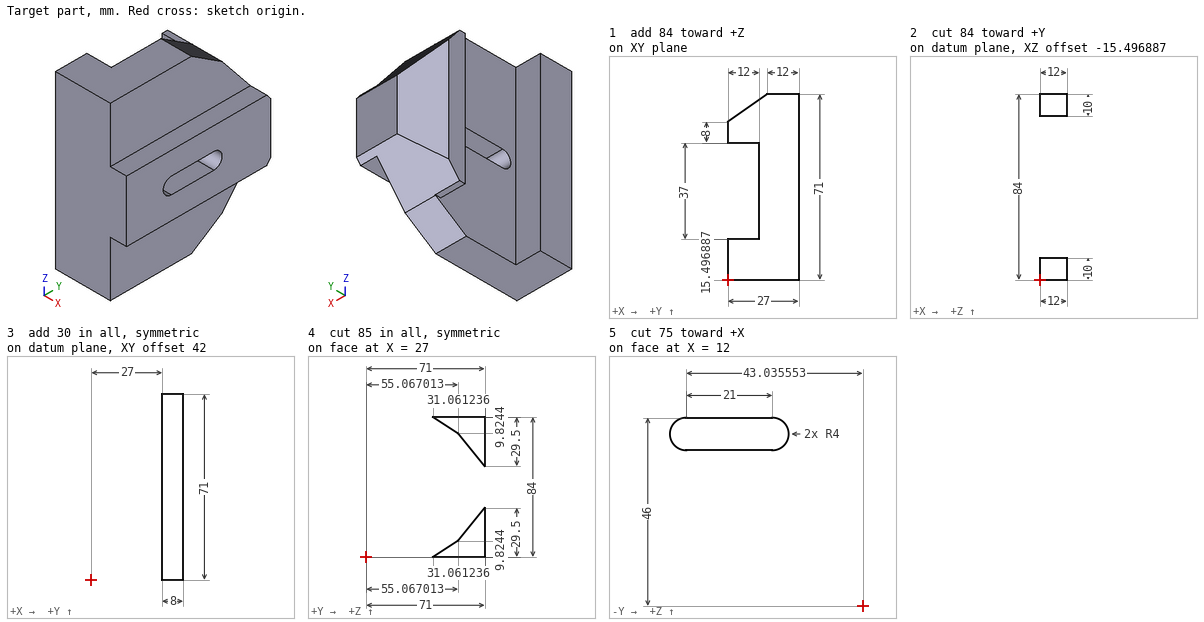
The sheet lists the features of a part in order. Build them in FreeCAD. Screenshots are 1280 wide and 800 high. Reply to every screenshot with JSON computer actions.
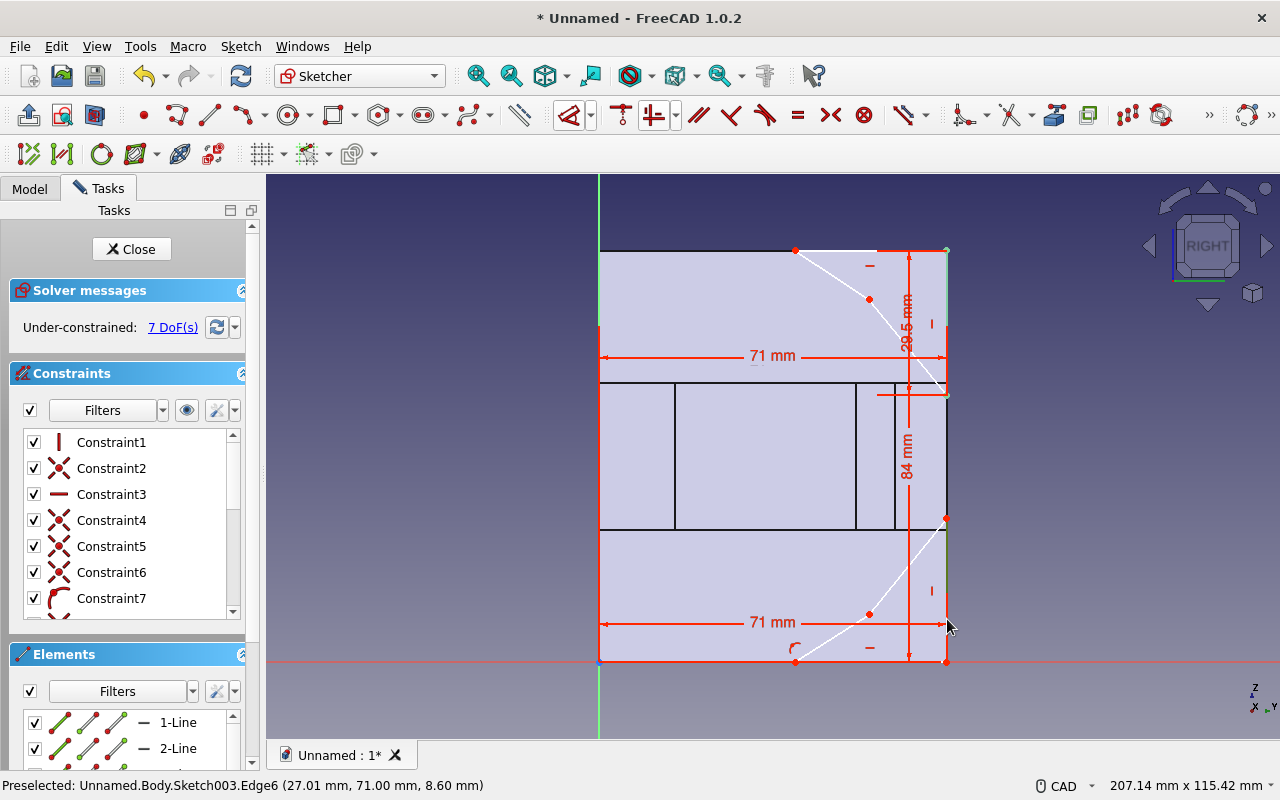
{"action": "key", "text": "i"}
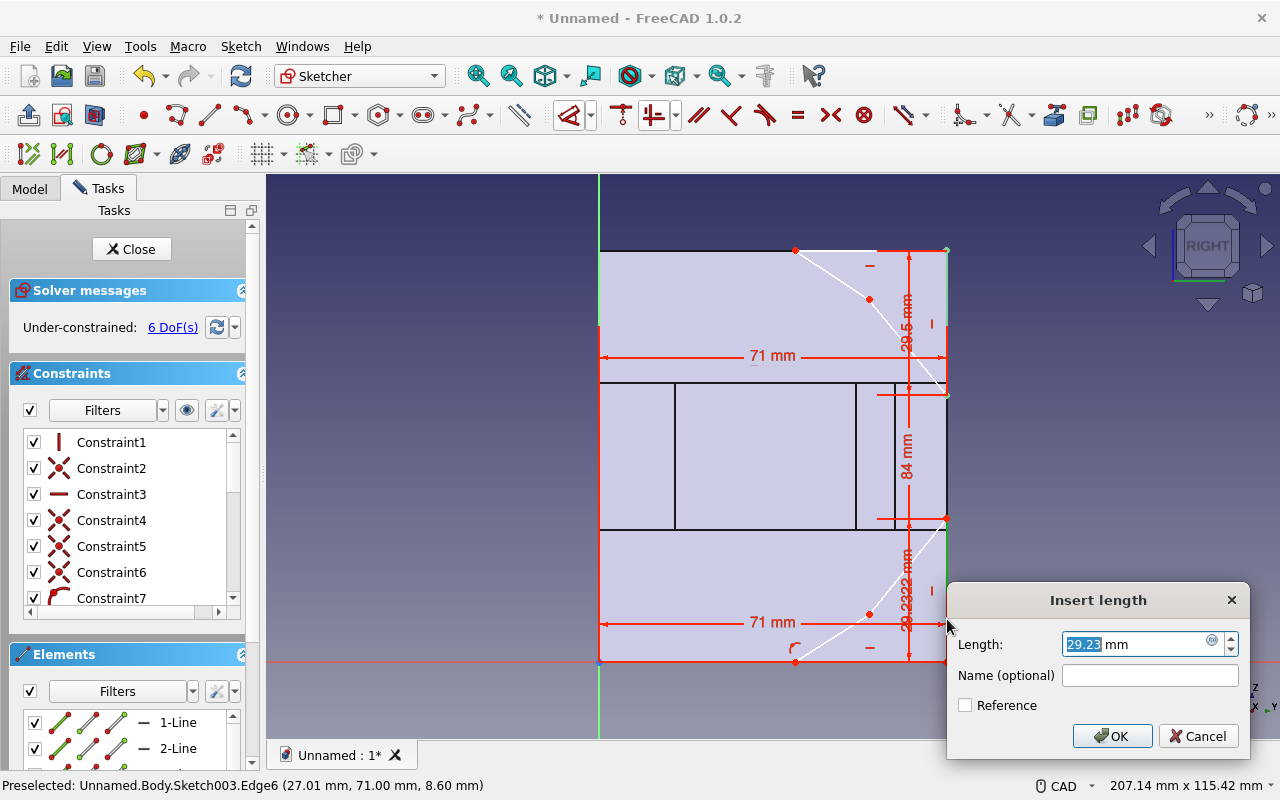
{"action": "type", "text": "29.5"}
{"action": "key", "text": "Return"}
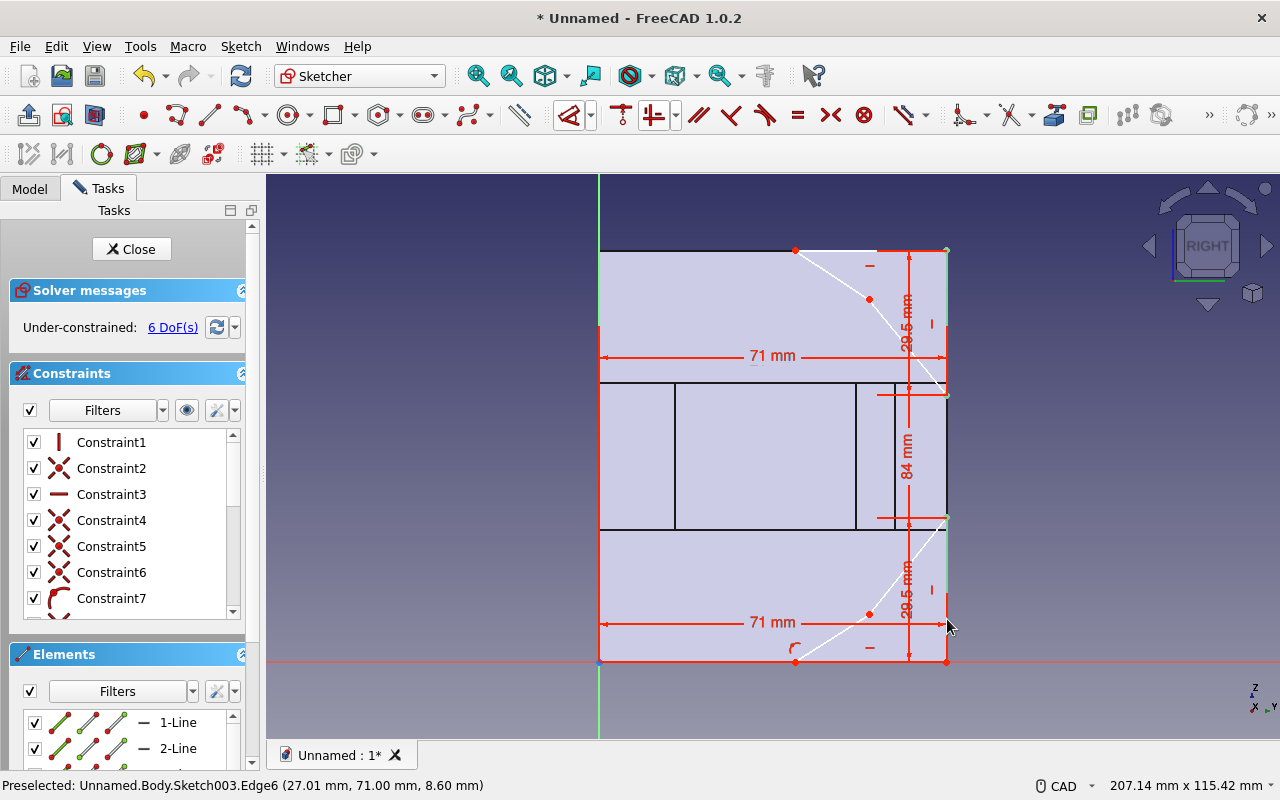
{"action": "left_click", "coordinate": [869, 615]}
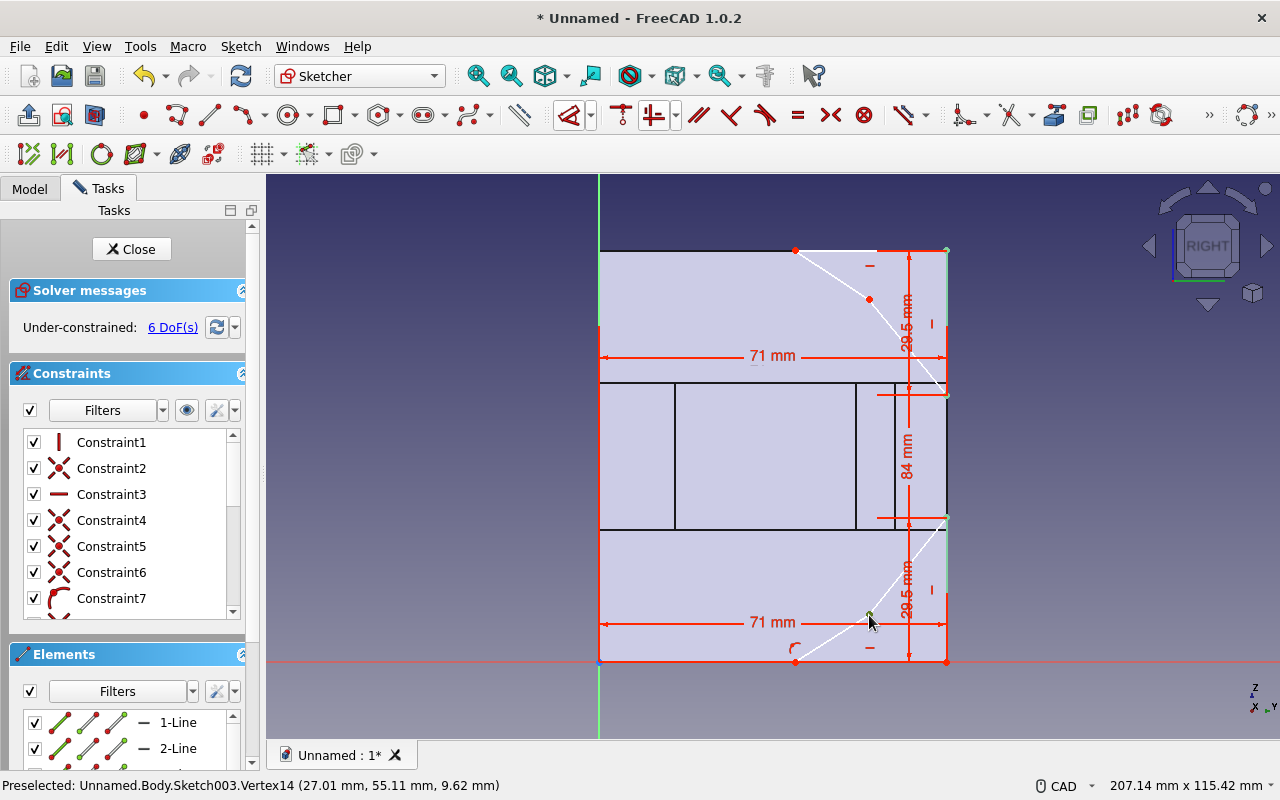
{"action": "left_click", "coordinate": [590, 116]}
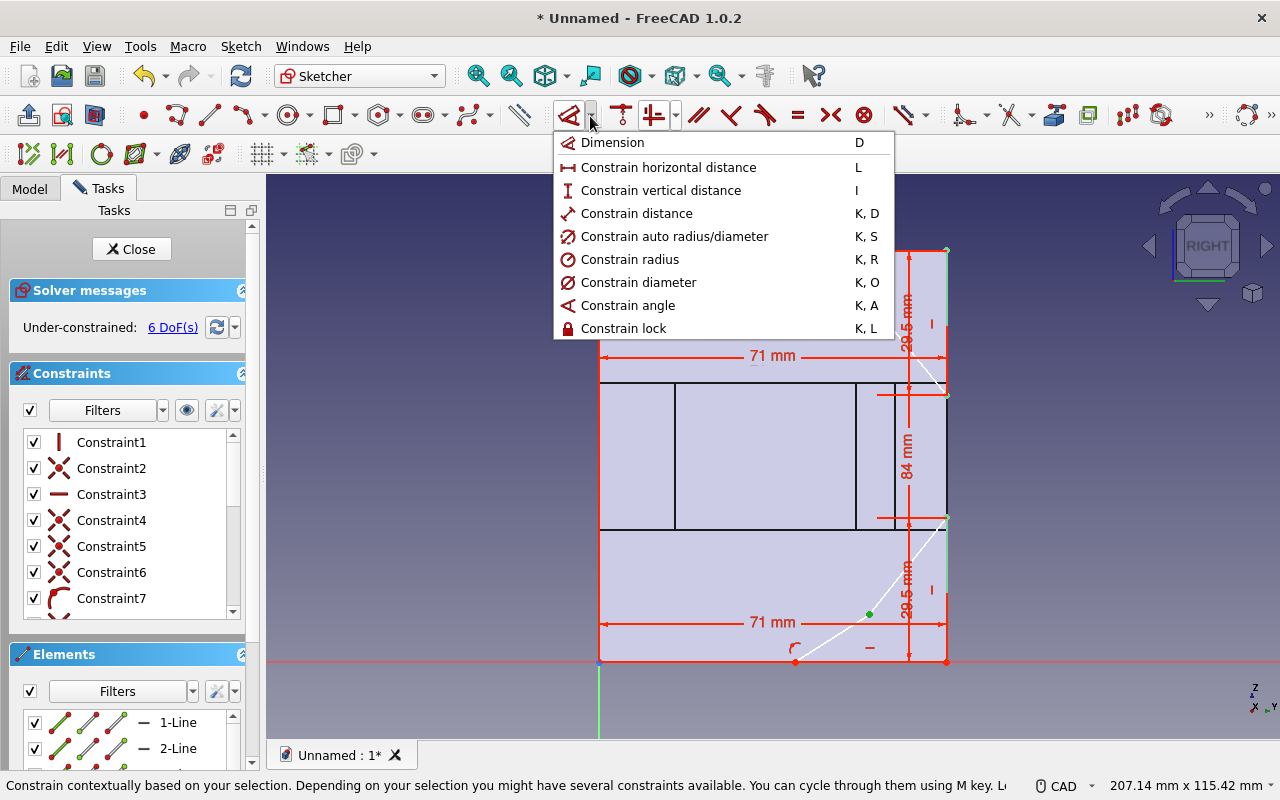
{"action": "left_click", "coordinate": [724, 190]}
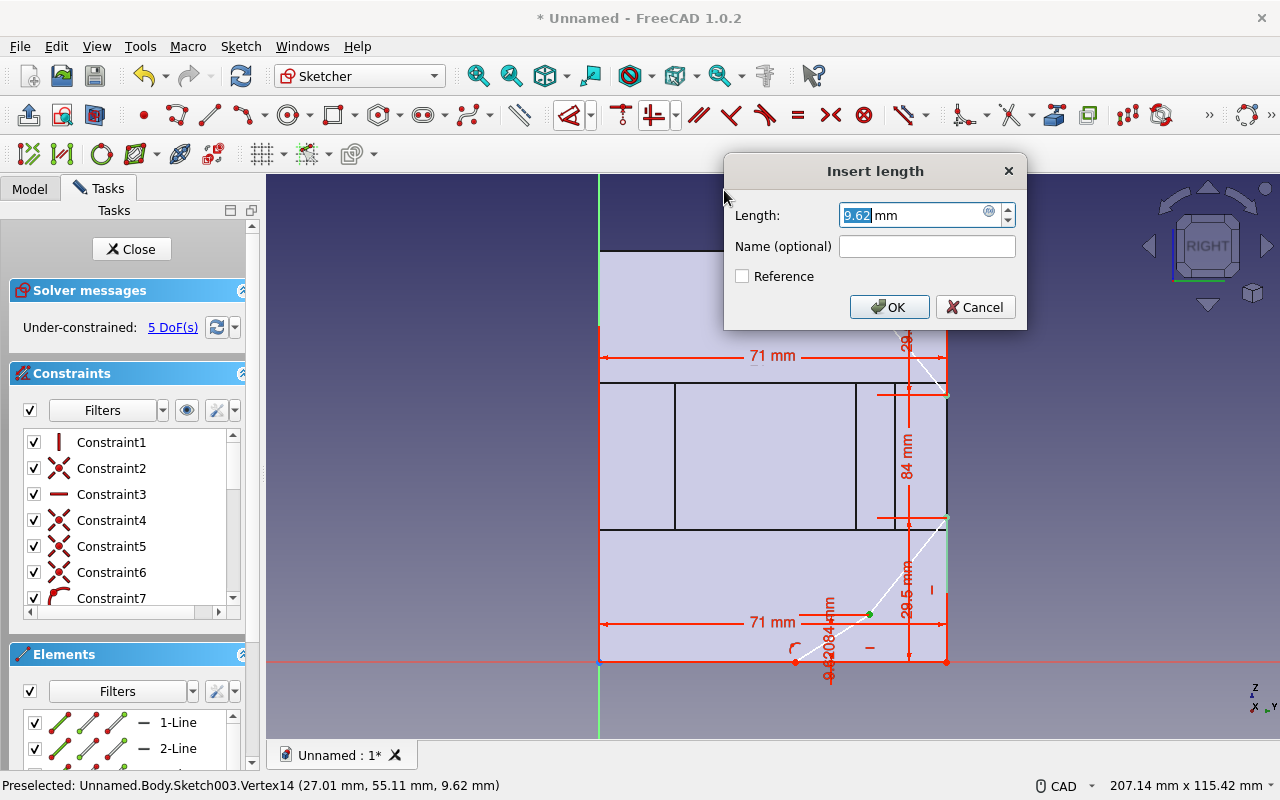
{"action": "type", "text": "9.8244"}
{"action": "key", "text": "Return"}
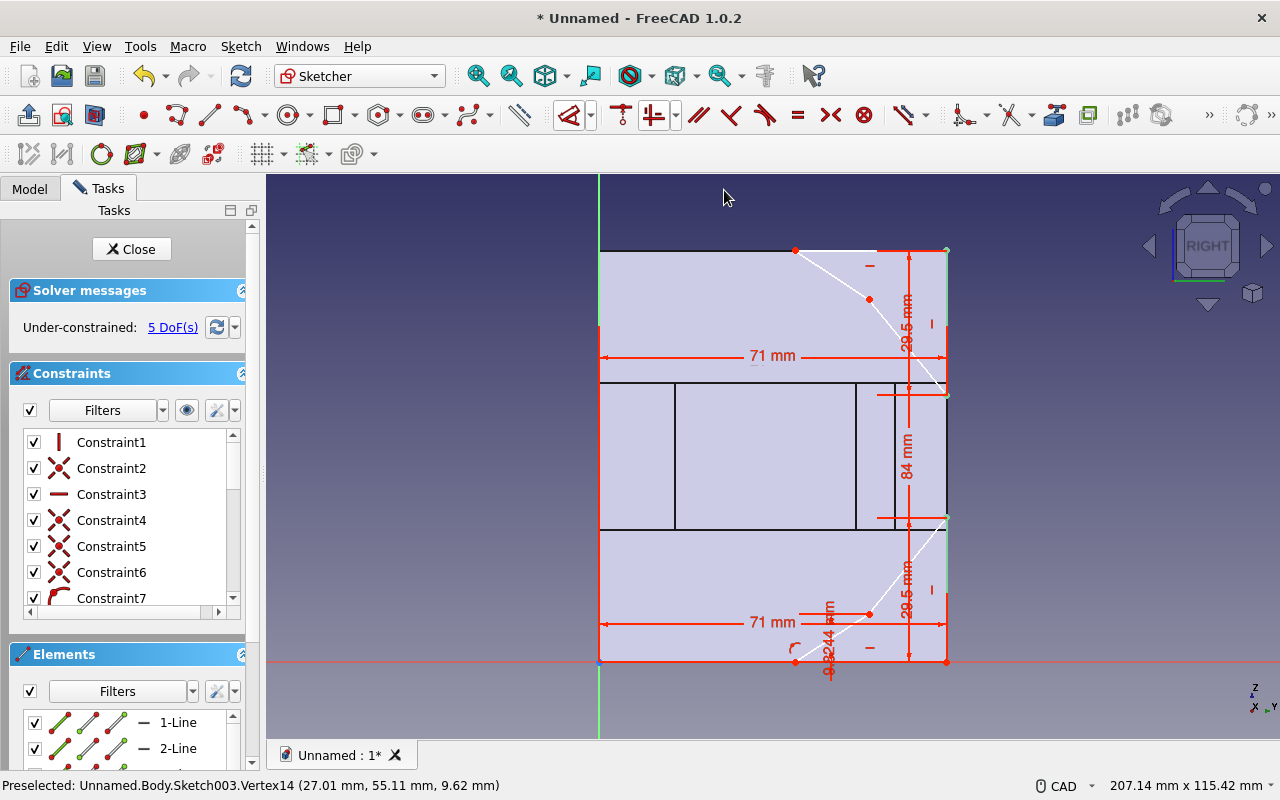
{"action": "left_click", "coordinate": [817, 266]}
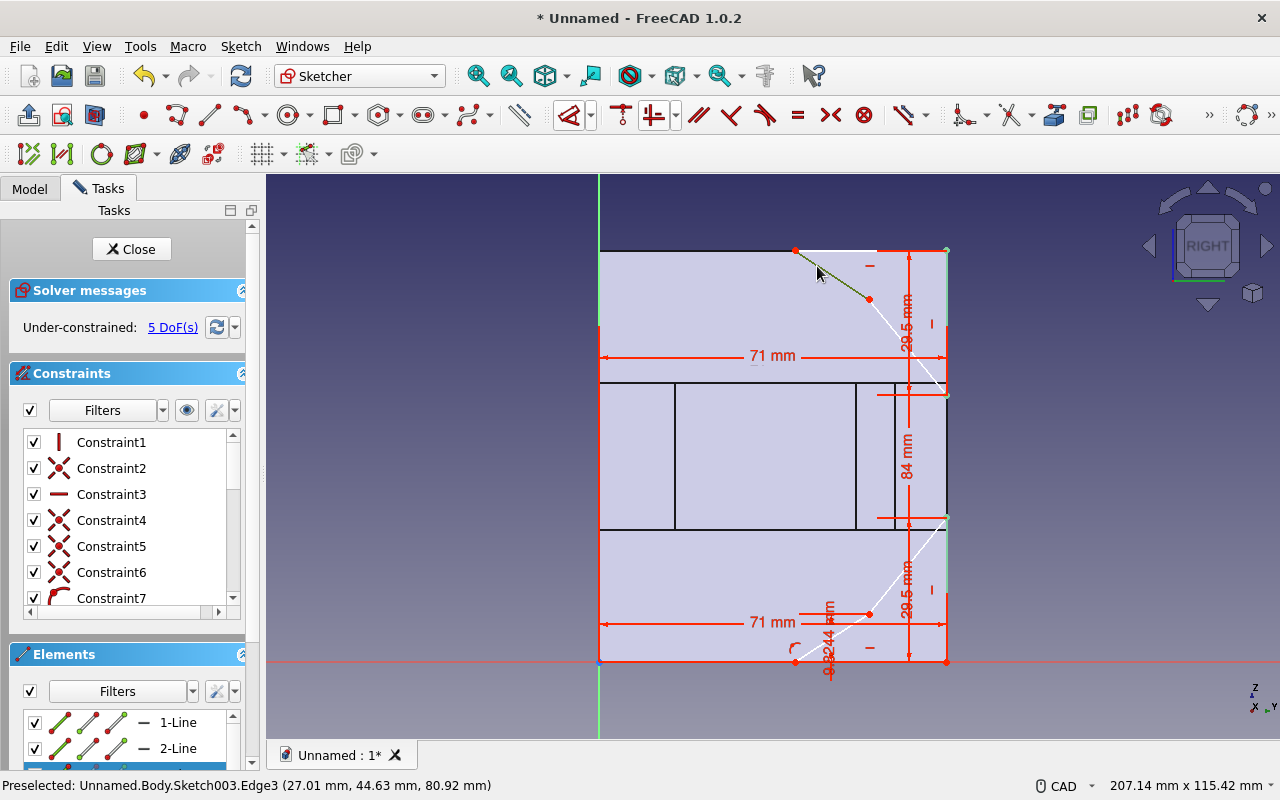
{"action": "left_click", "coordinate": [590, 116]}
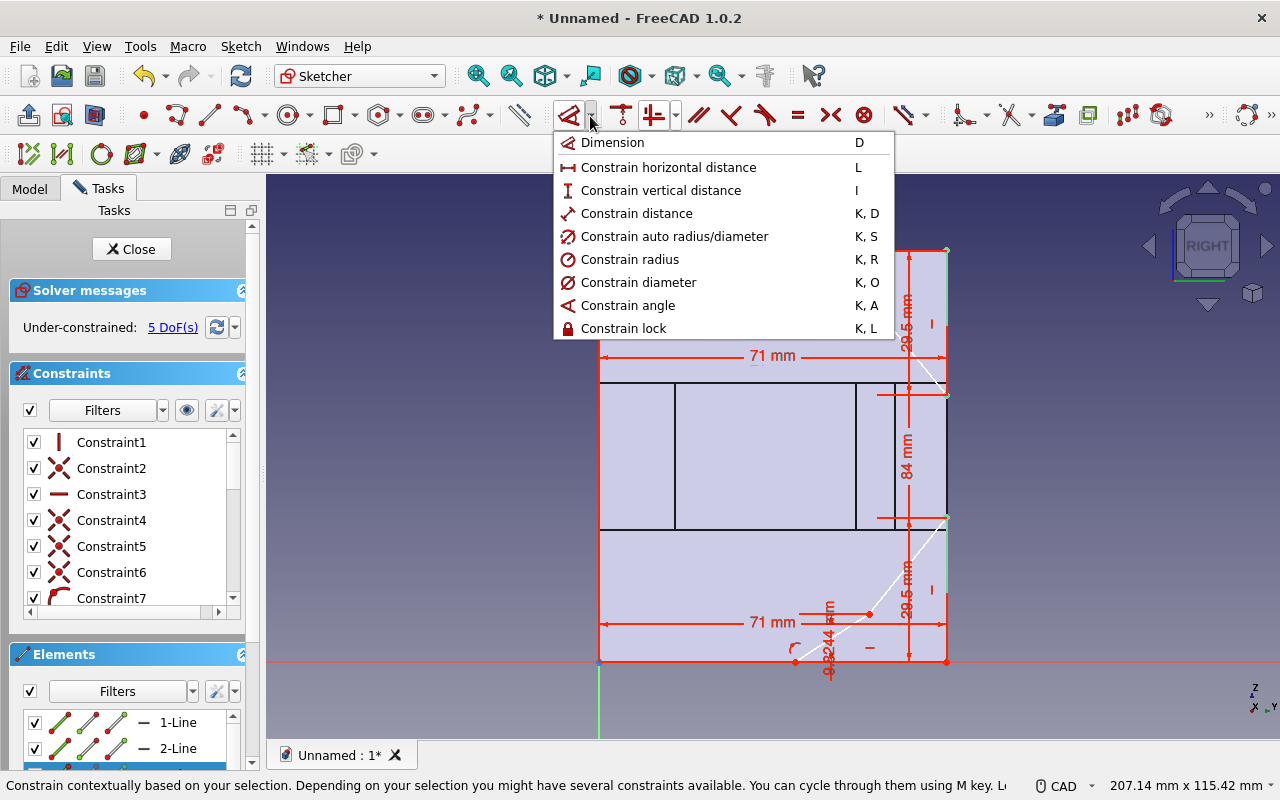
{"action": "left_click", "coordinate": [724, 190]}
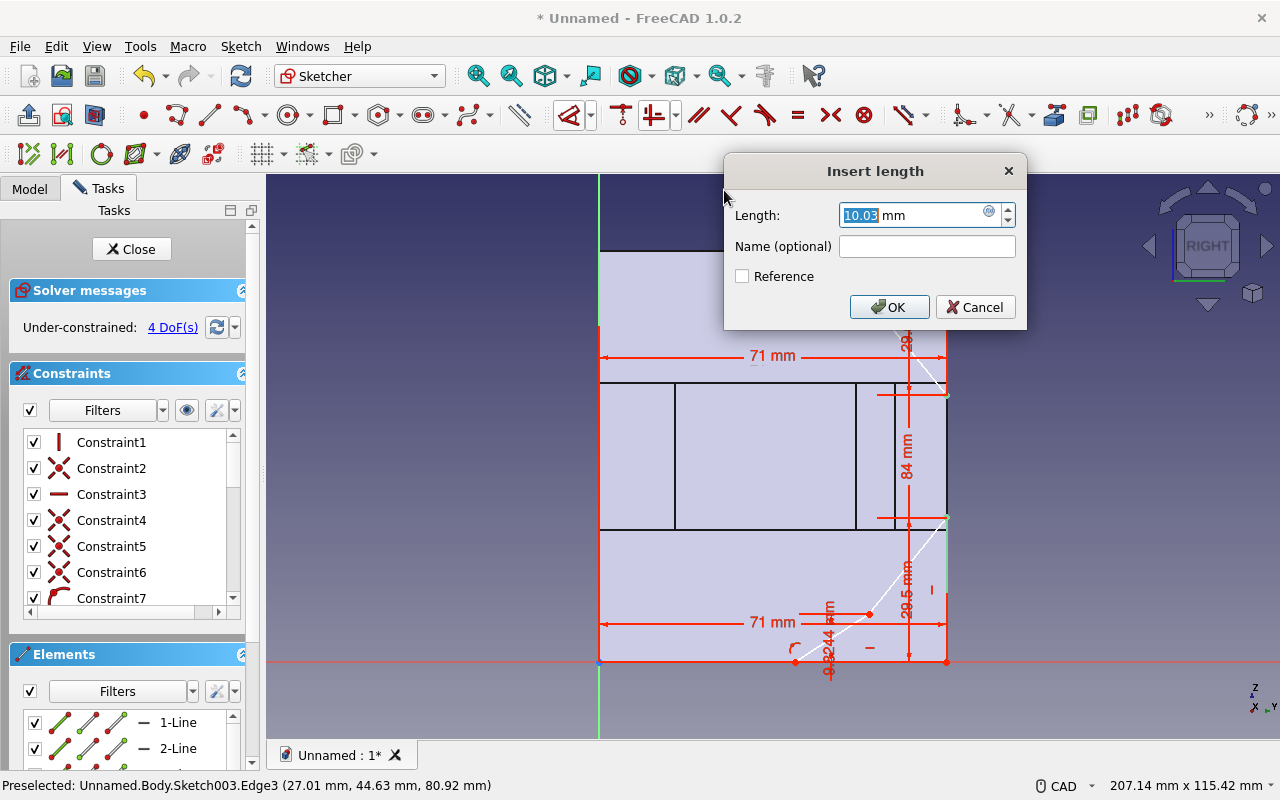
{"action": "type", "text": "9.8244"}
{"action": "key", "text": "Return"}